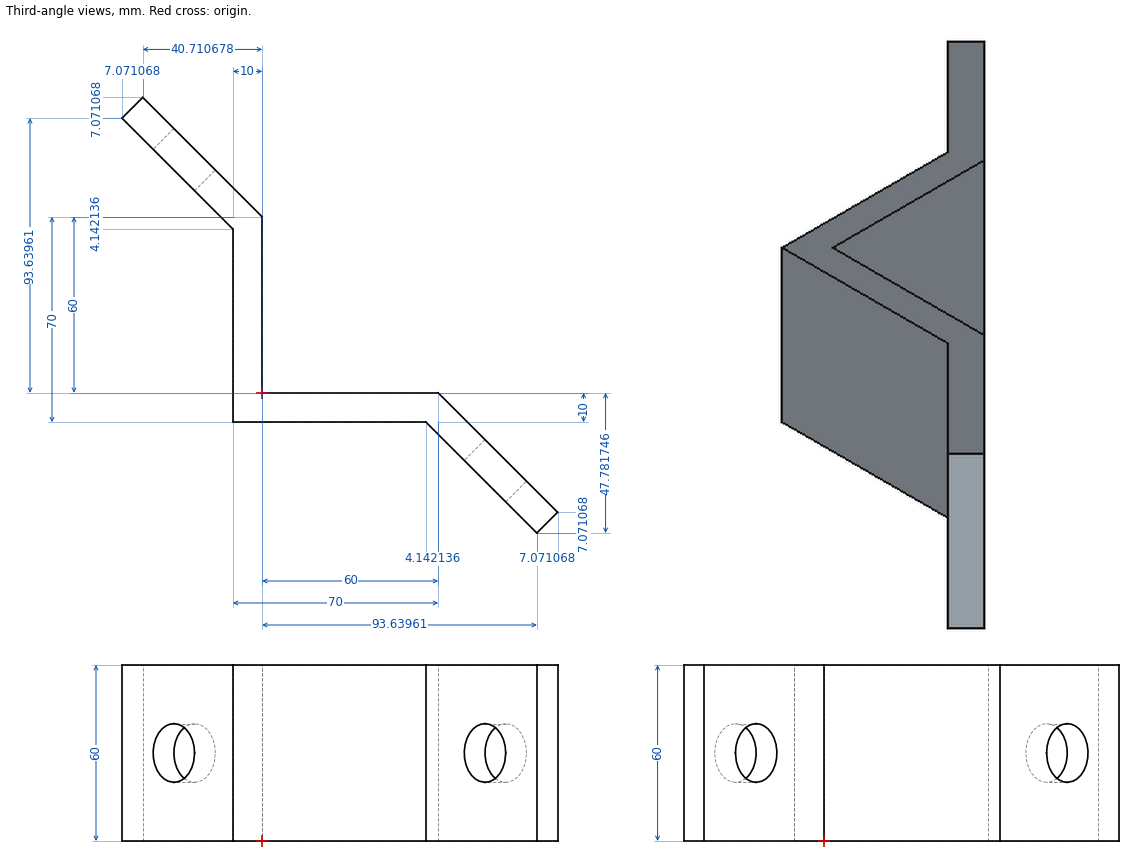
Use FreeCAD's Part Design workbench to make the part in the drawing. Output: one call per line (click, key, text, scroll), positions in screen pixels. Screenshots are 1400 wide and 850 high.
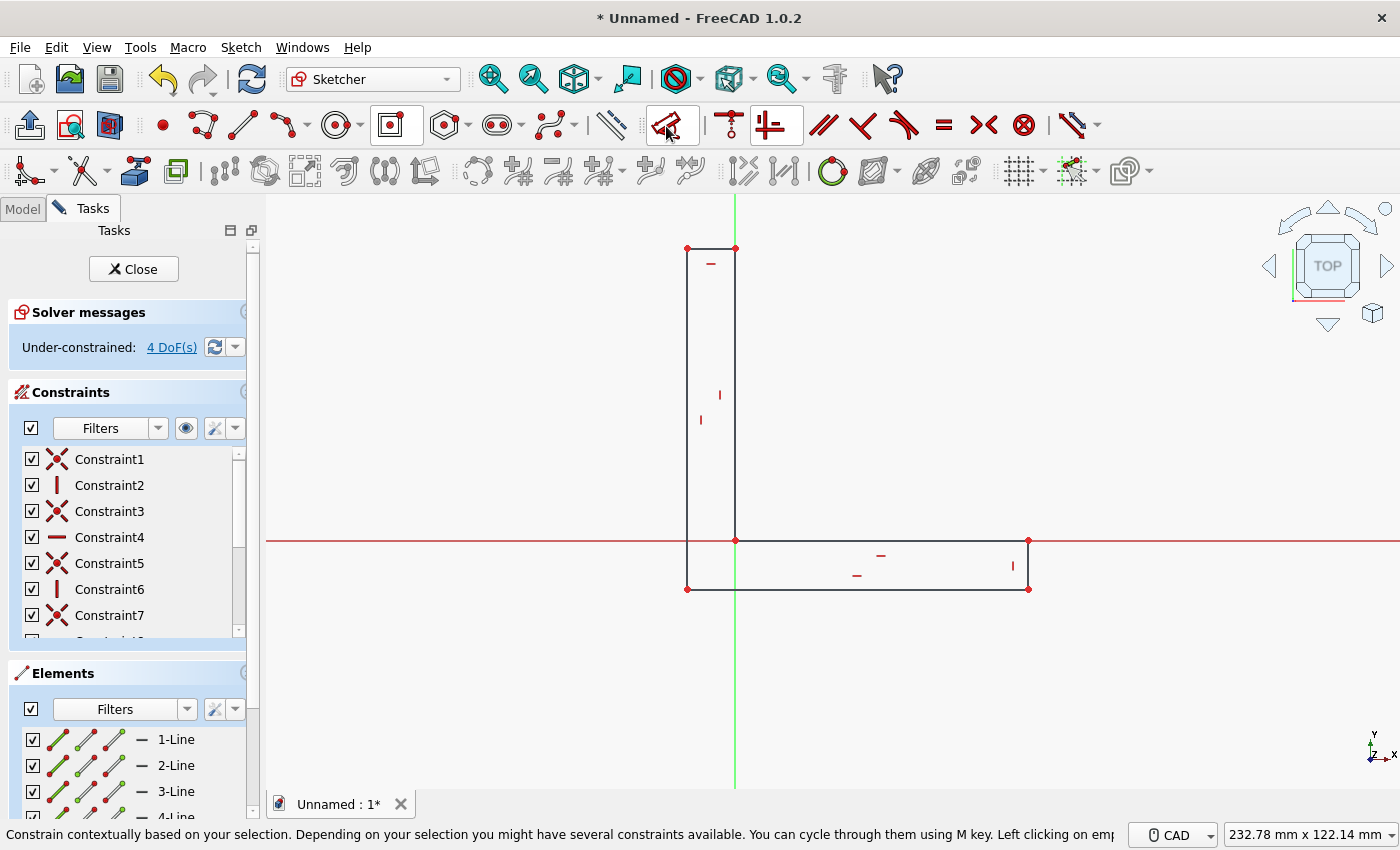
click(735, 453)
click(701, 395)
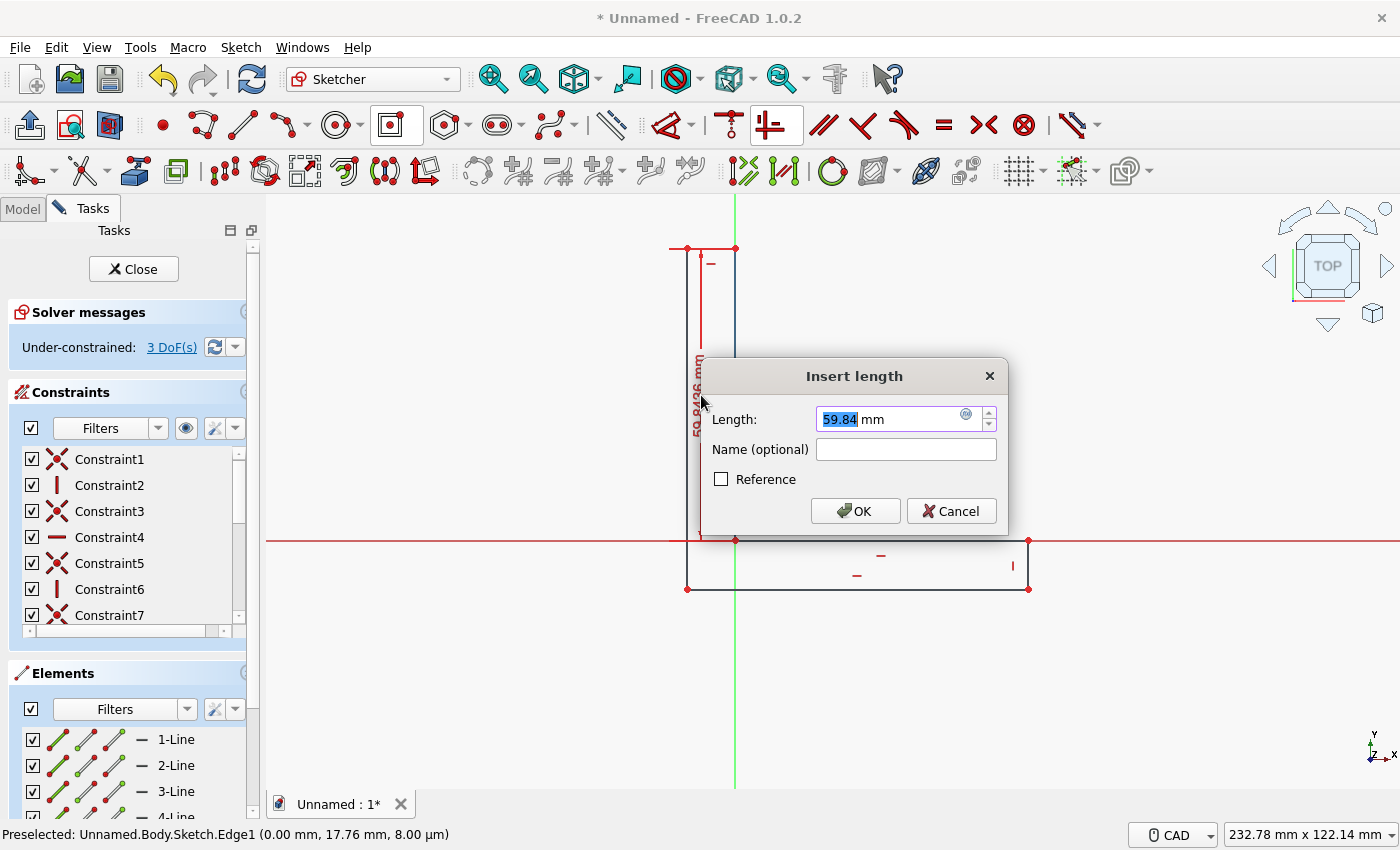
text(60)
key(Return)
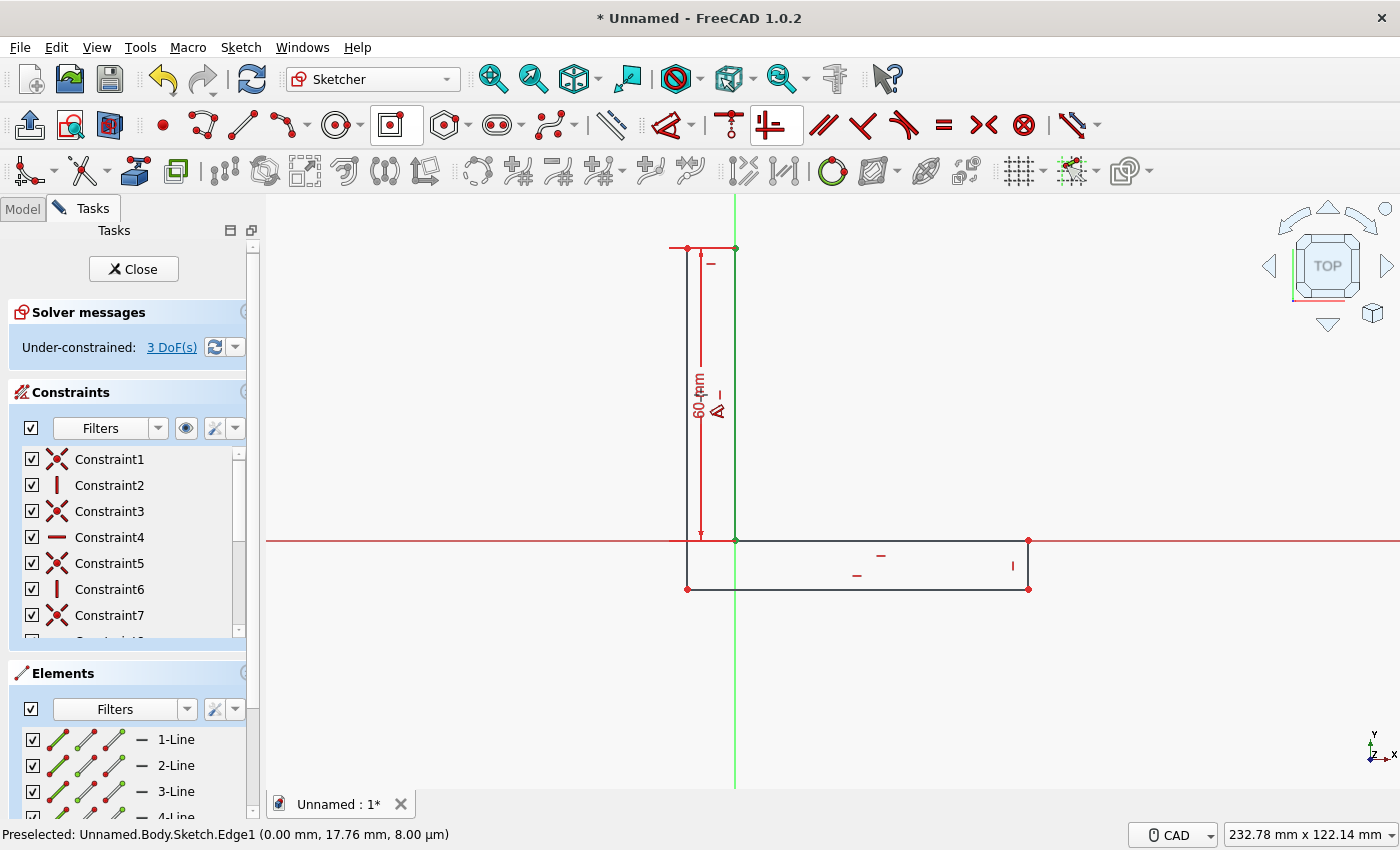
click(721, 248)
click(711, 282)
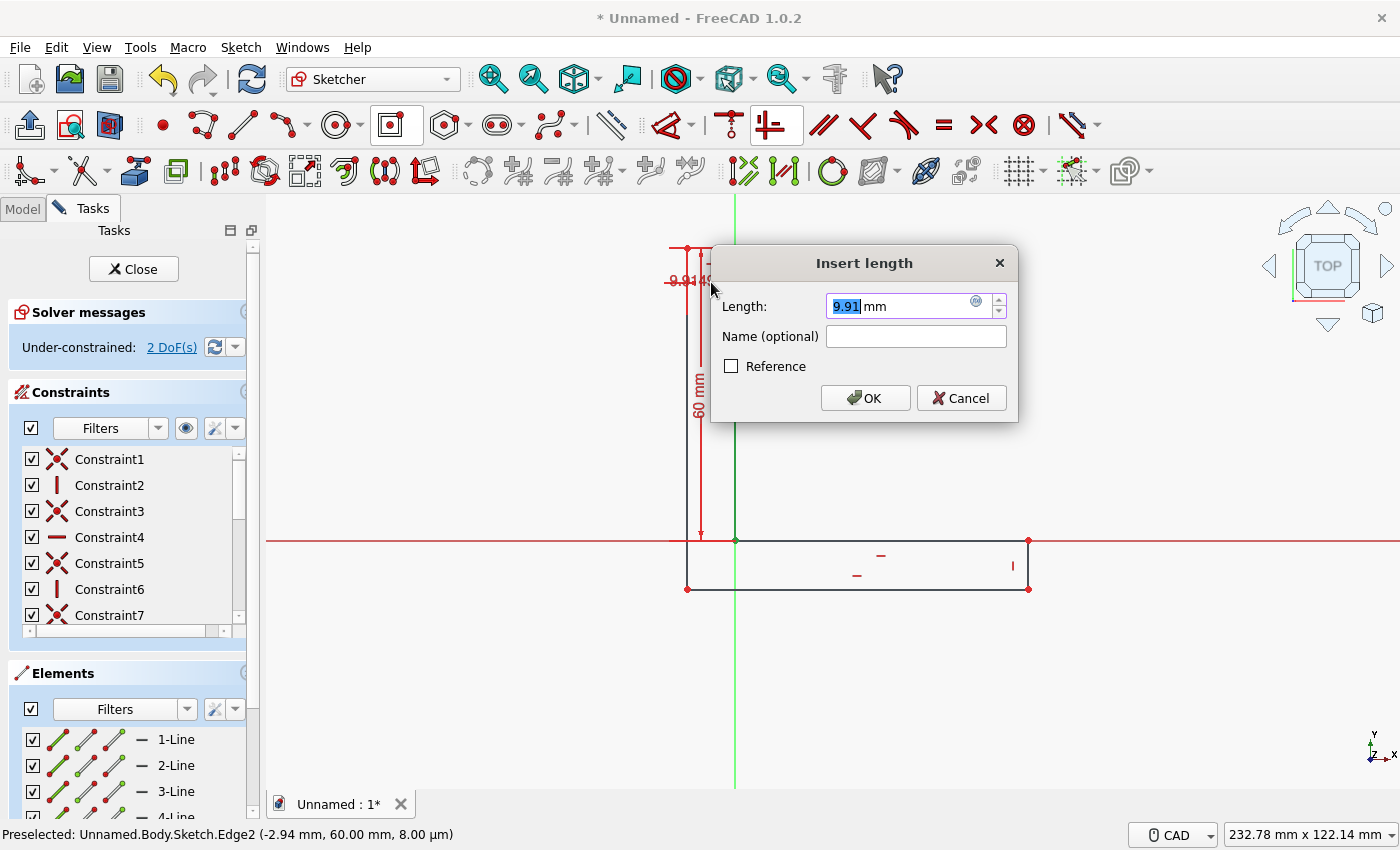
text(10)
key(Return)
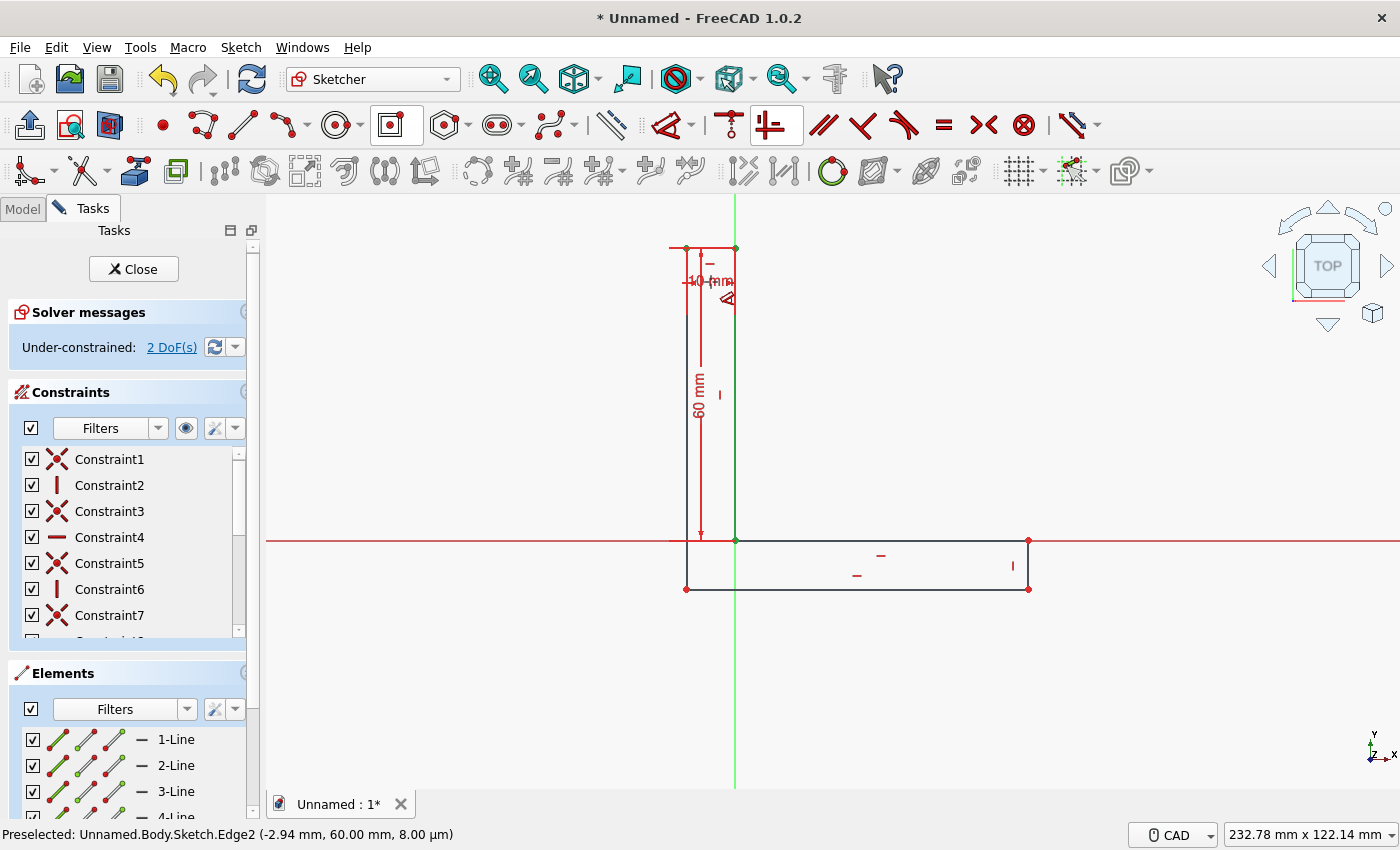
click(687, 351)
click(653, 419)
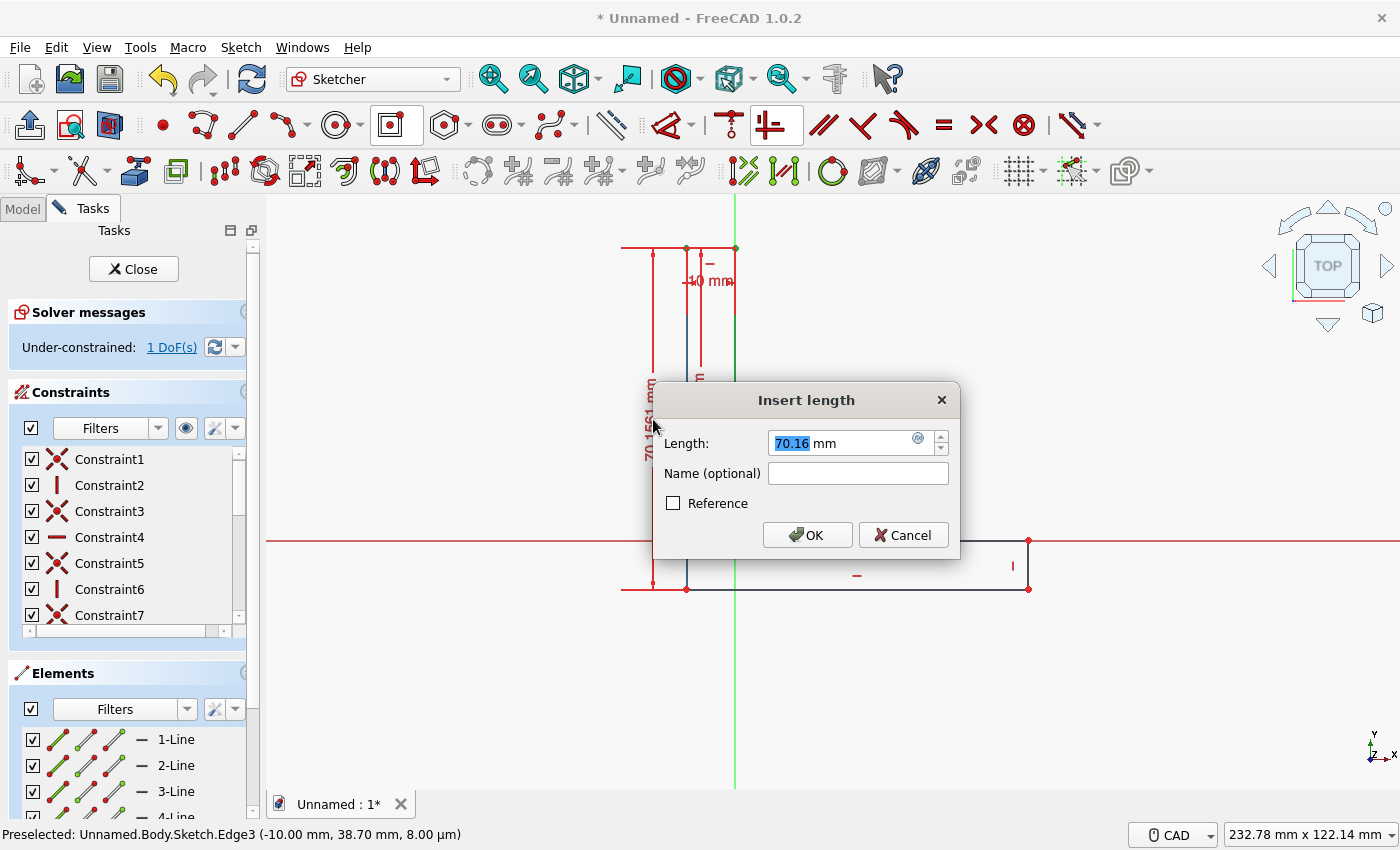
text(70)
key(Return)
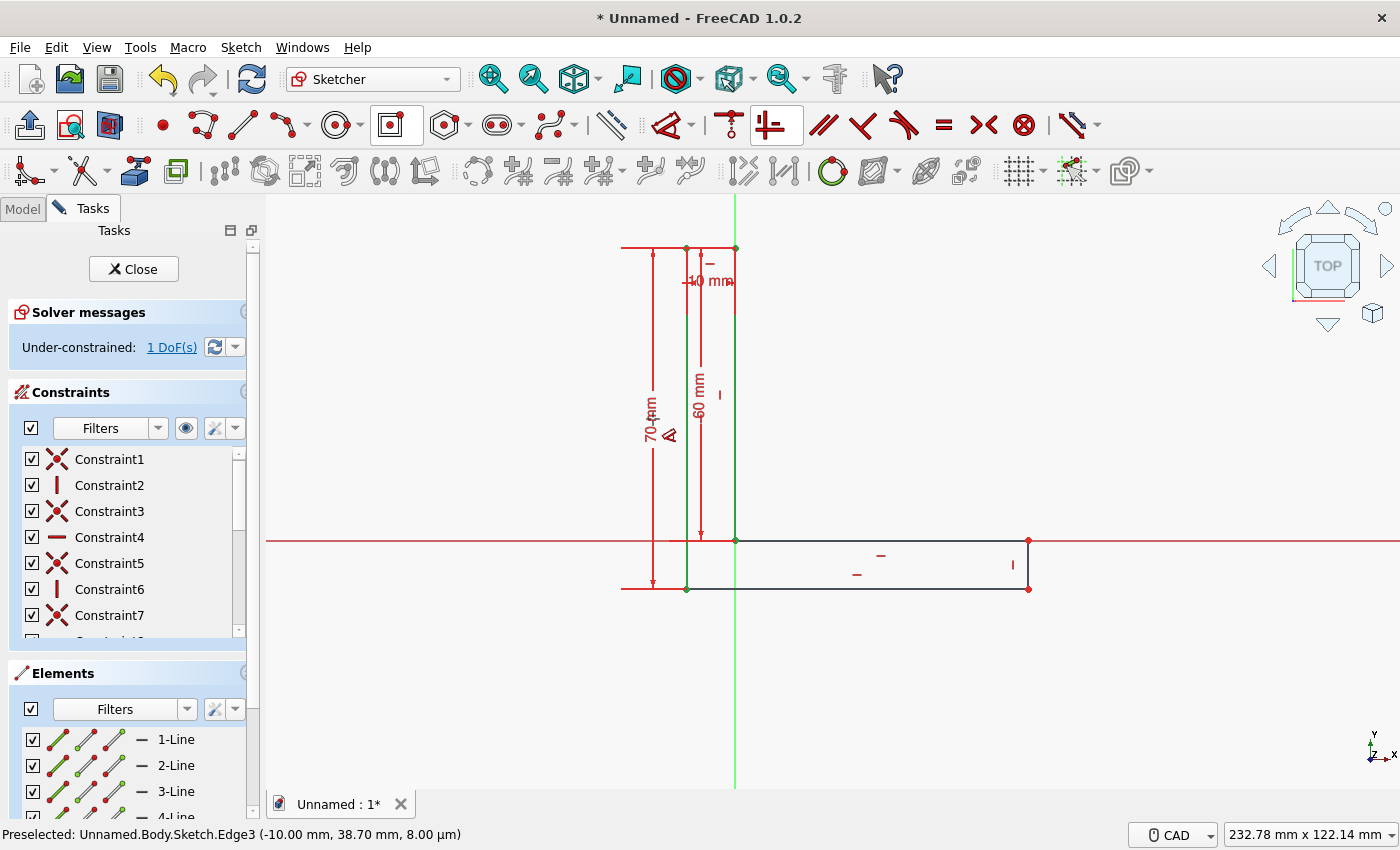
click(789, 589)
click(857, 623)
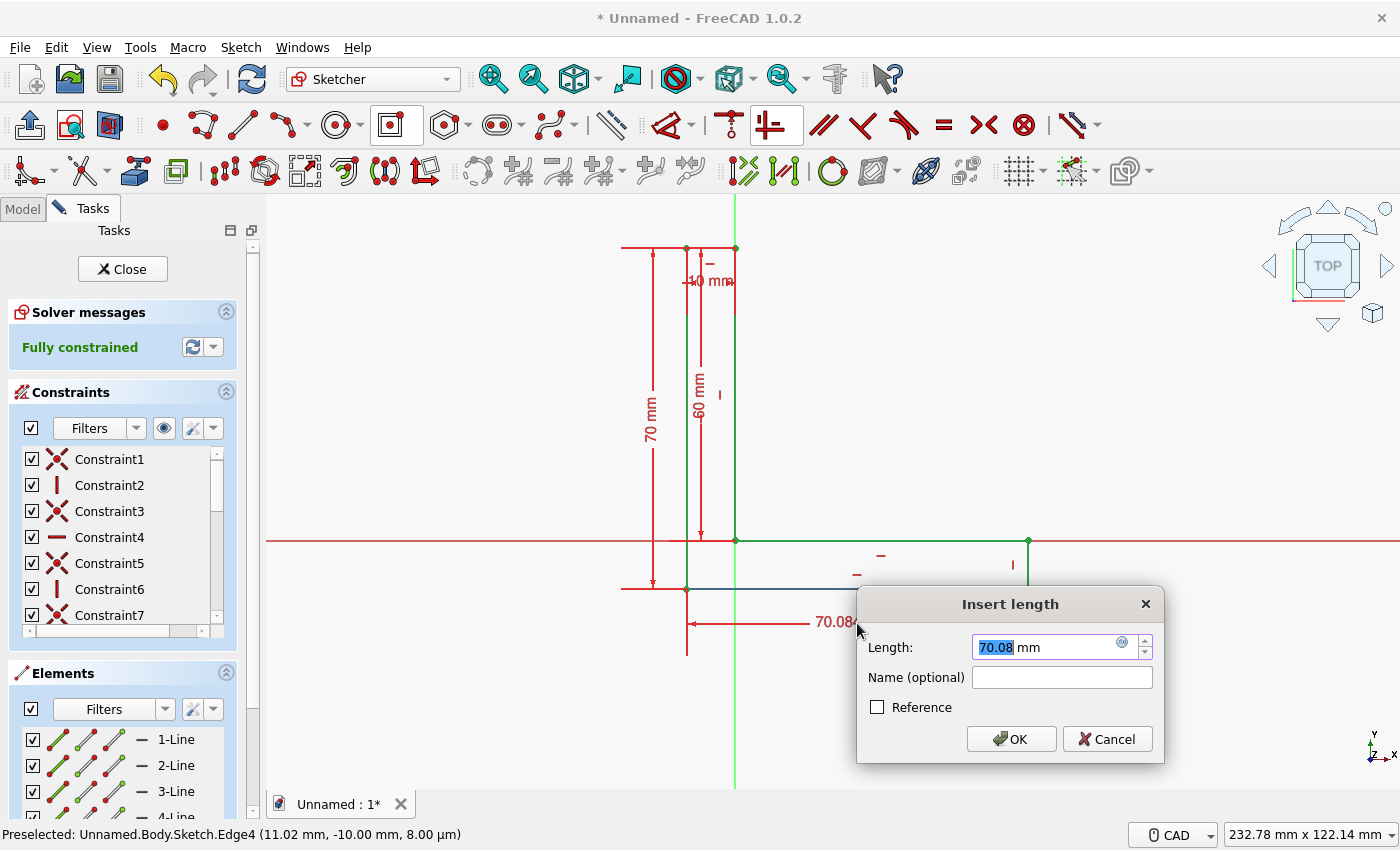
text(70)
key(Return)
key(Escape)